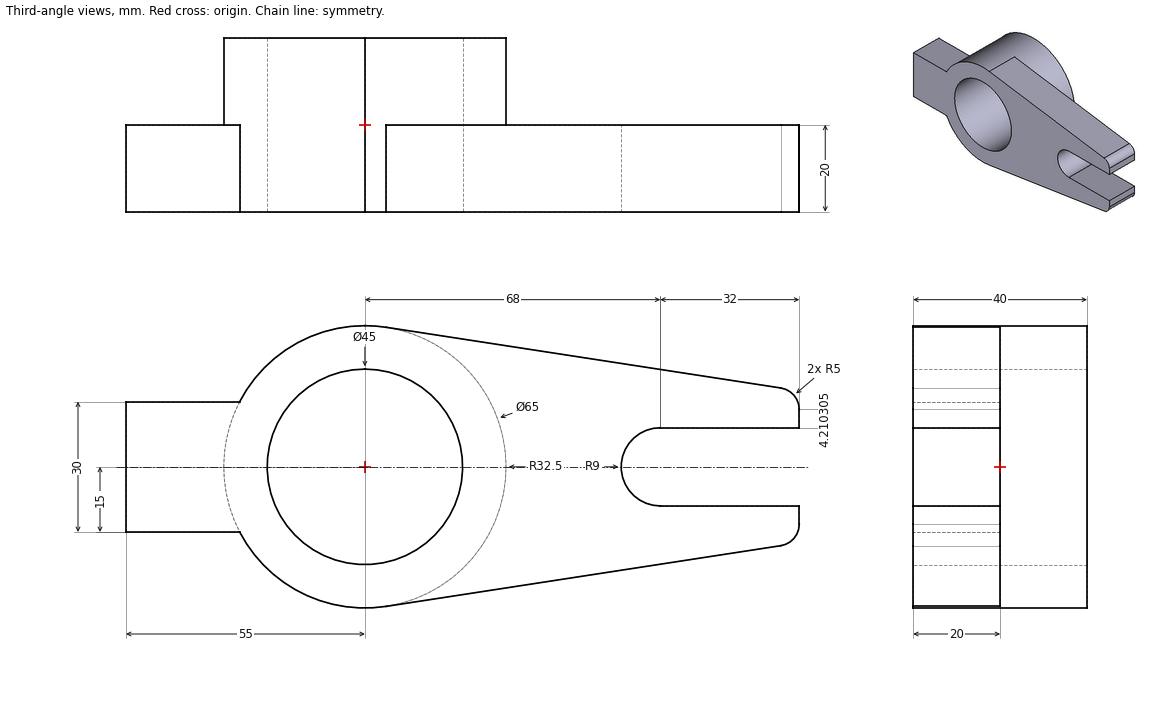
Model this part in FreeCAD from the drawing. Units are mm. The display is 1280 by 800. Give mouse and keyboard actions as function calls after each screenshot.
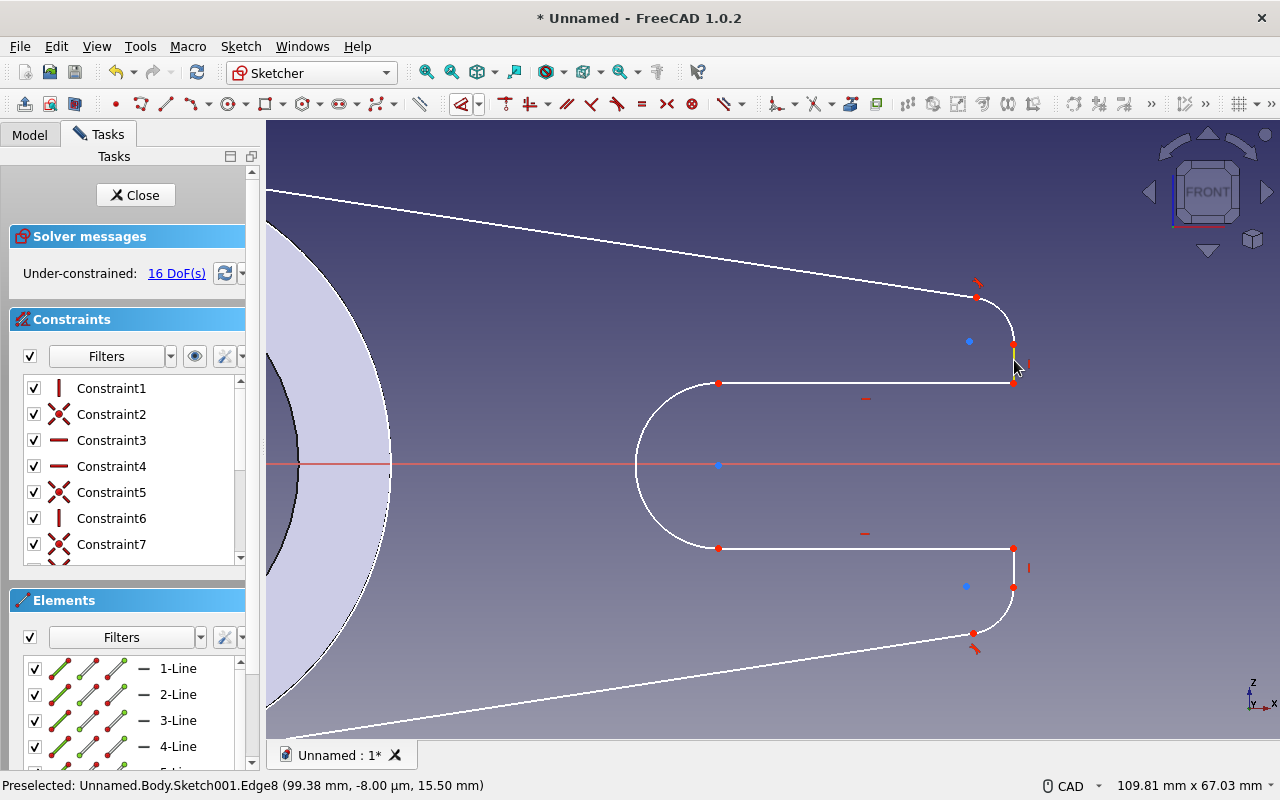
click(1014, 360)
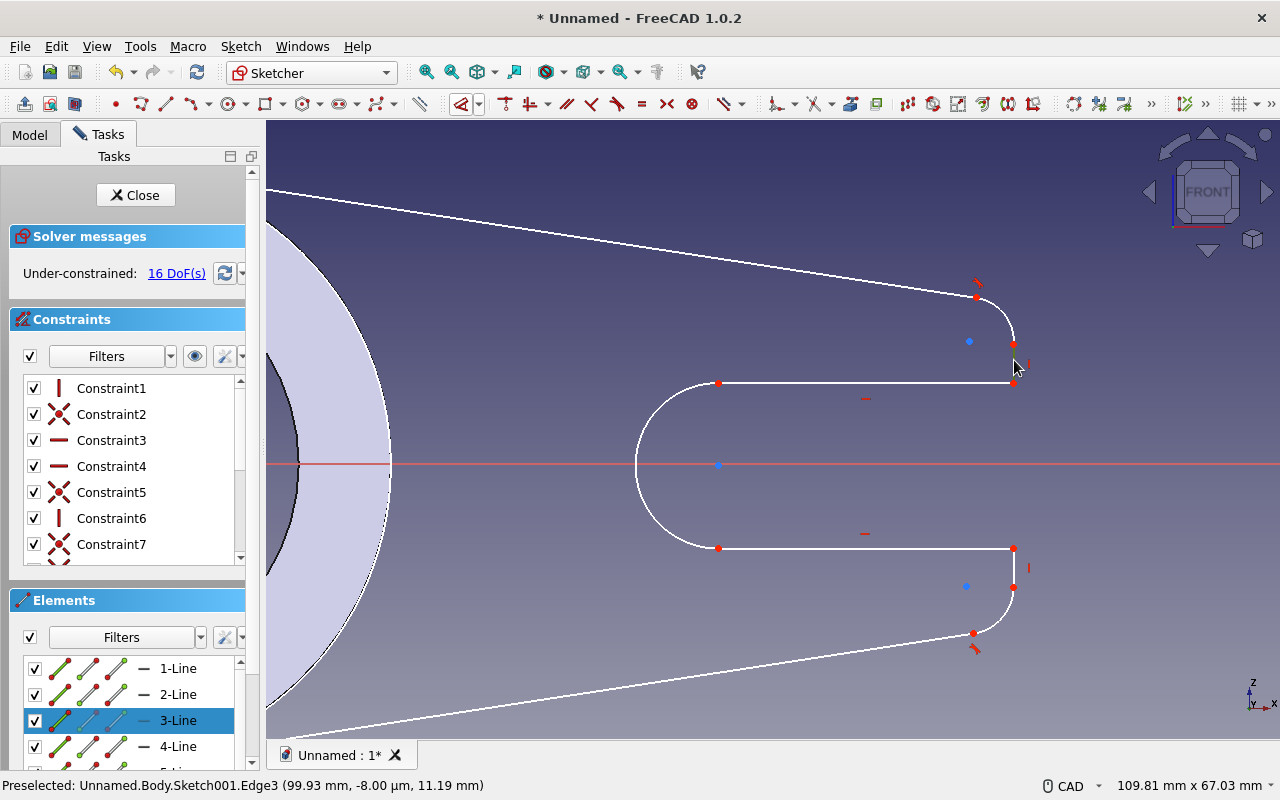
click(1011, 325)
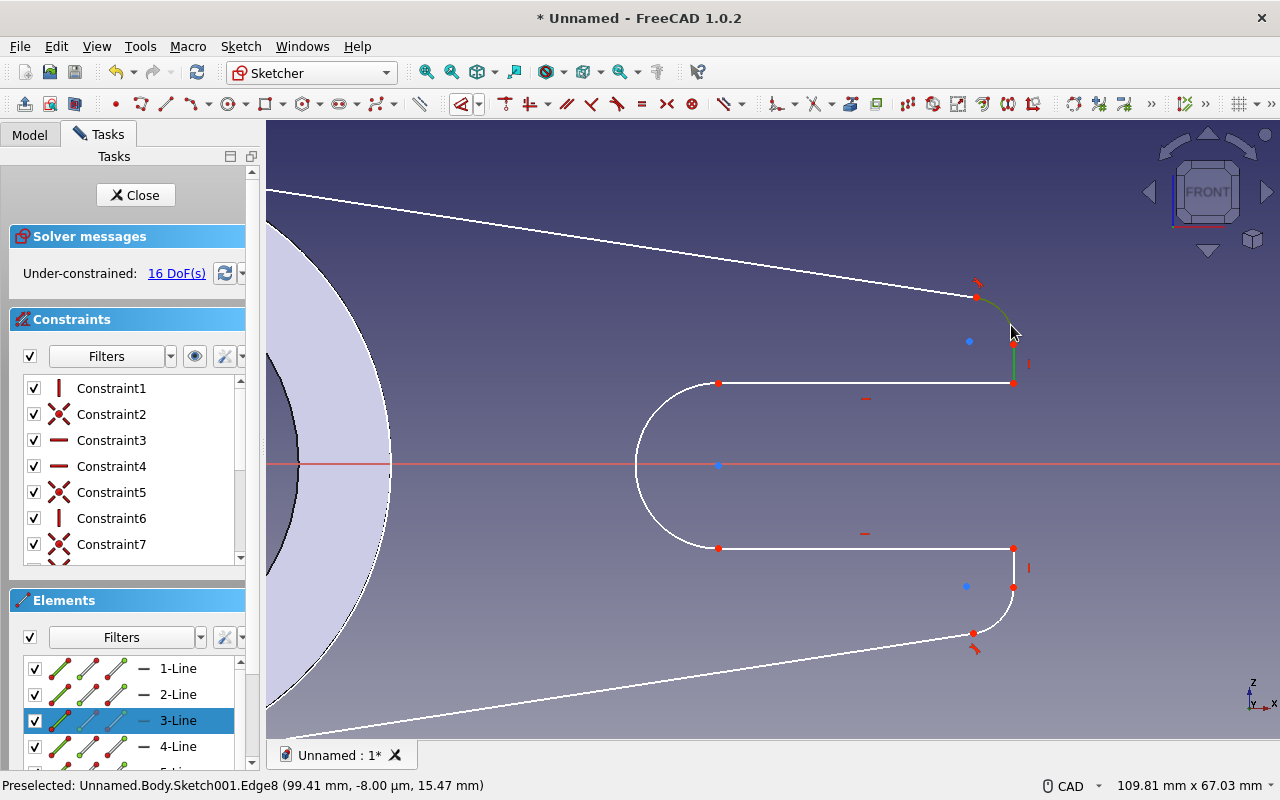
key(t)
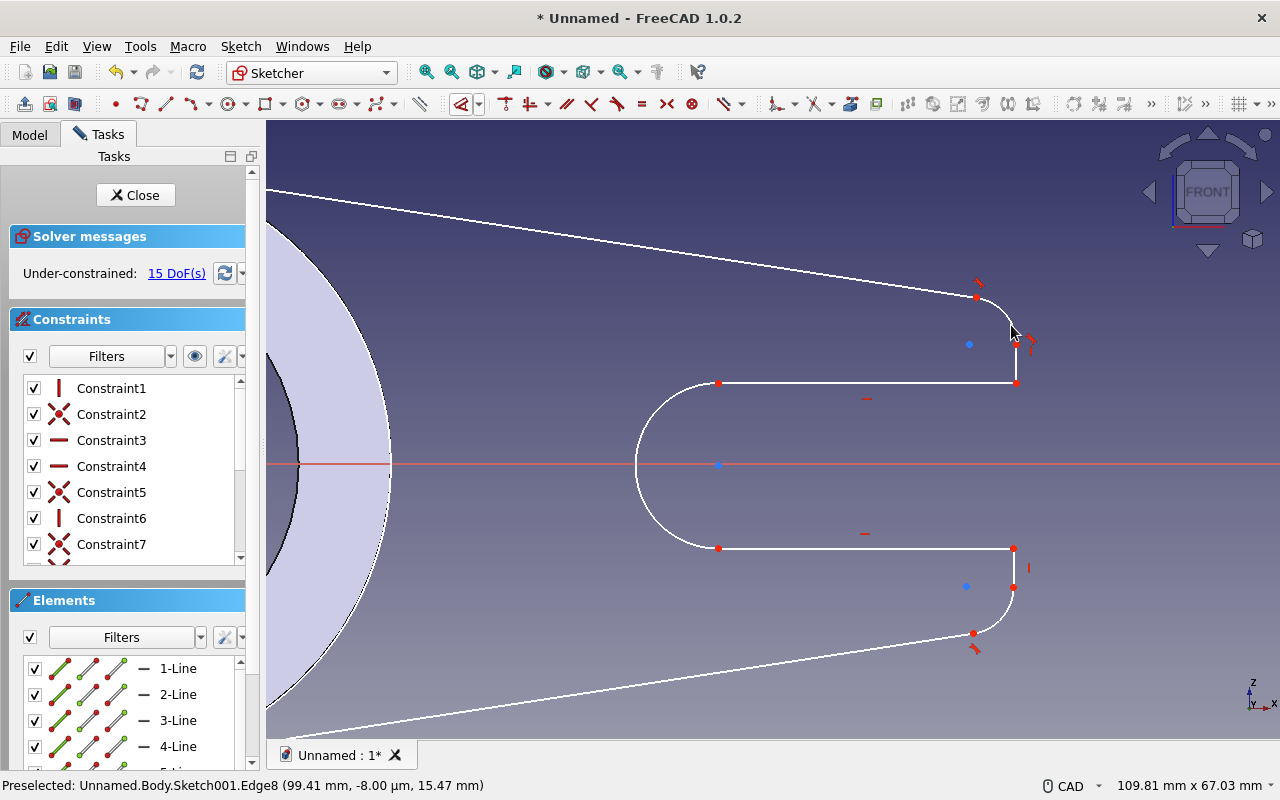
click(927, 383)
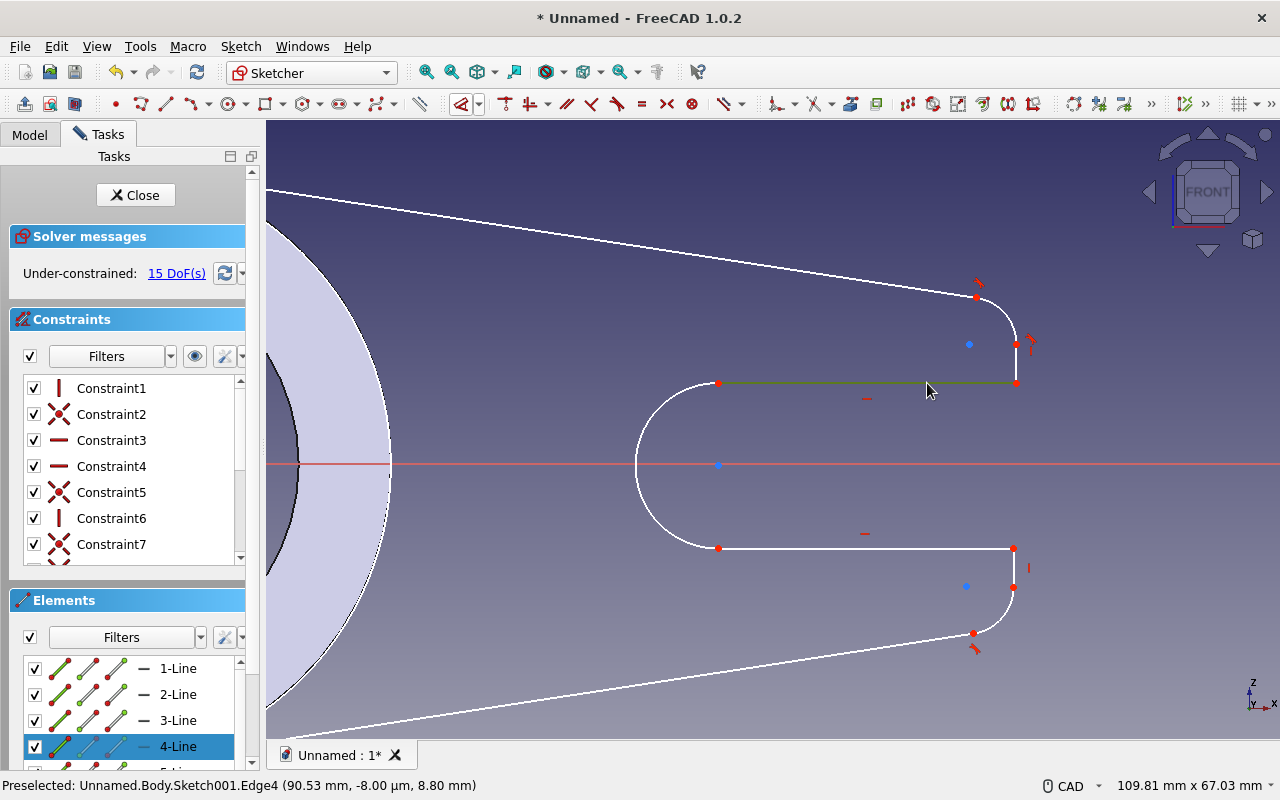
click(651, 417)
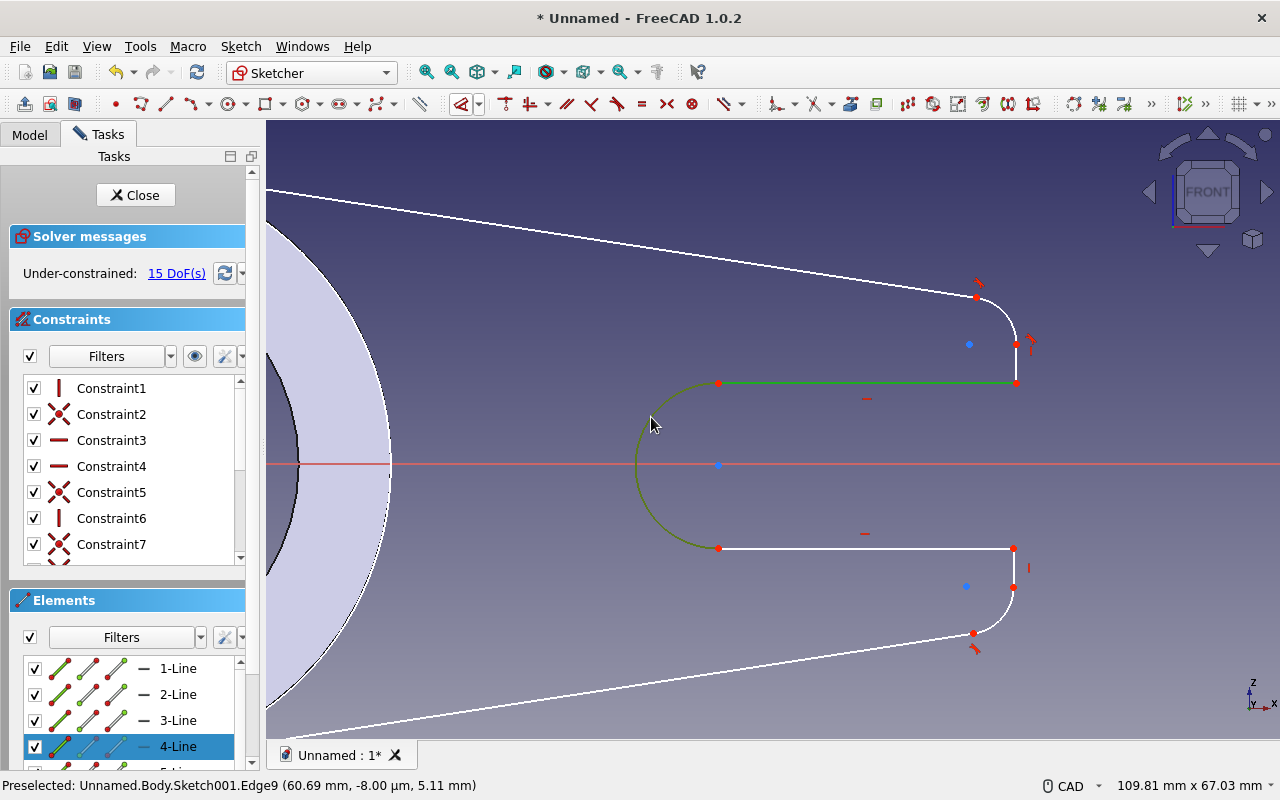
click(617, 104)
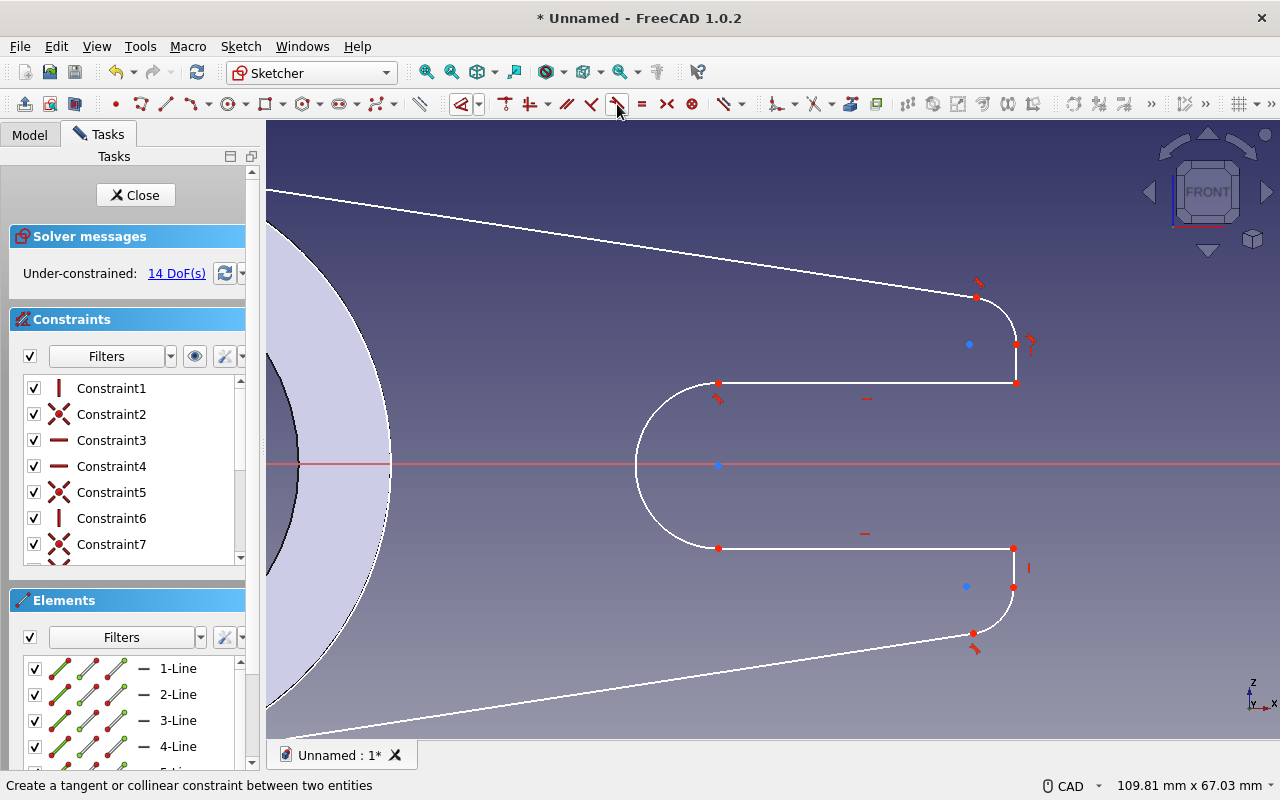
click(807, 549)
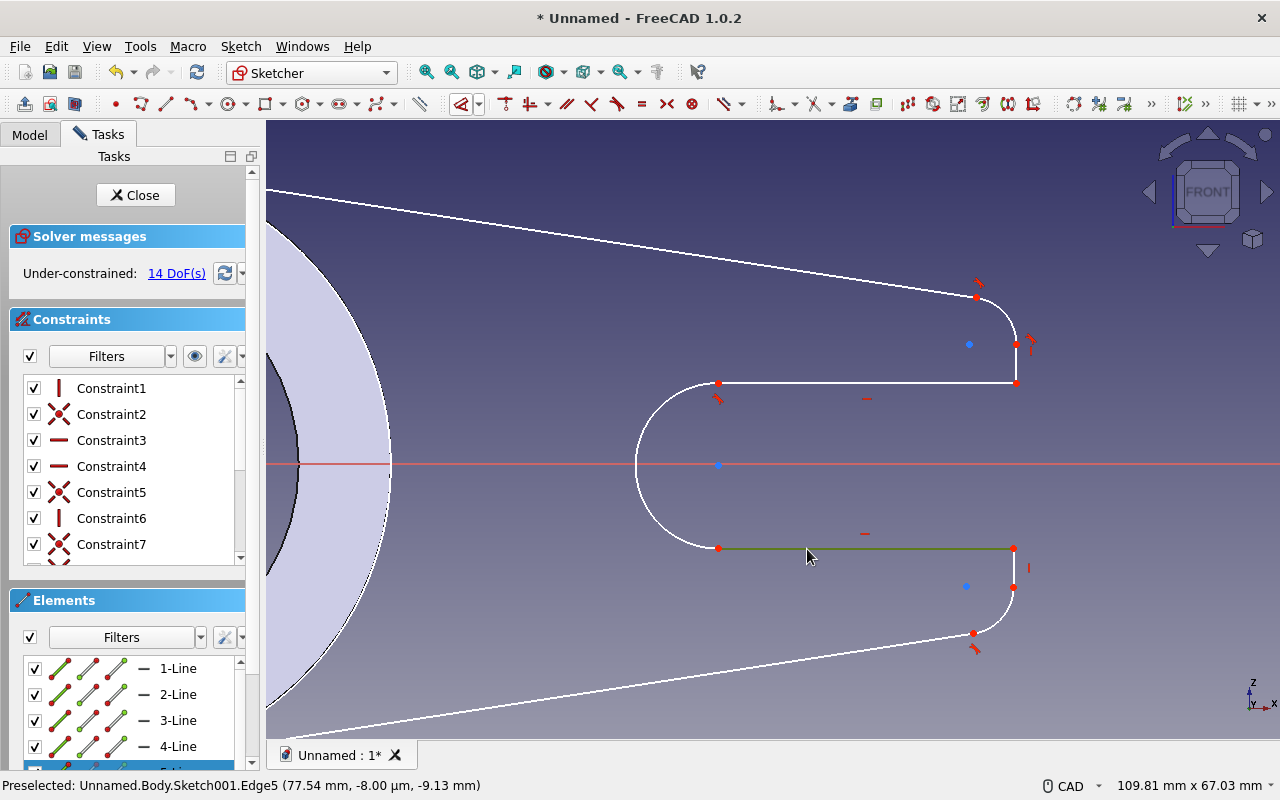
click(651, 417)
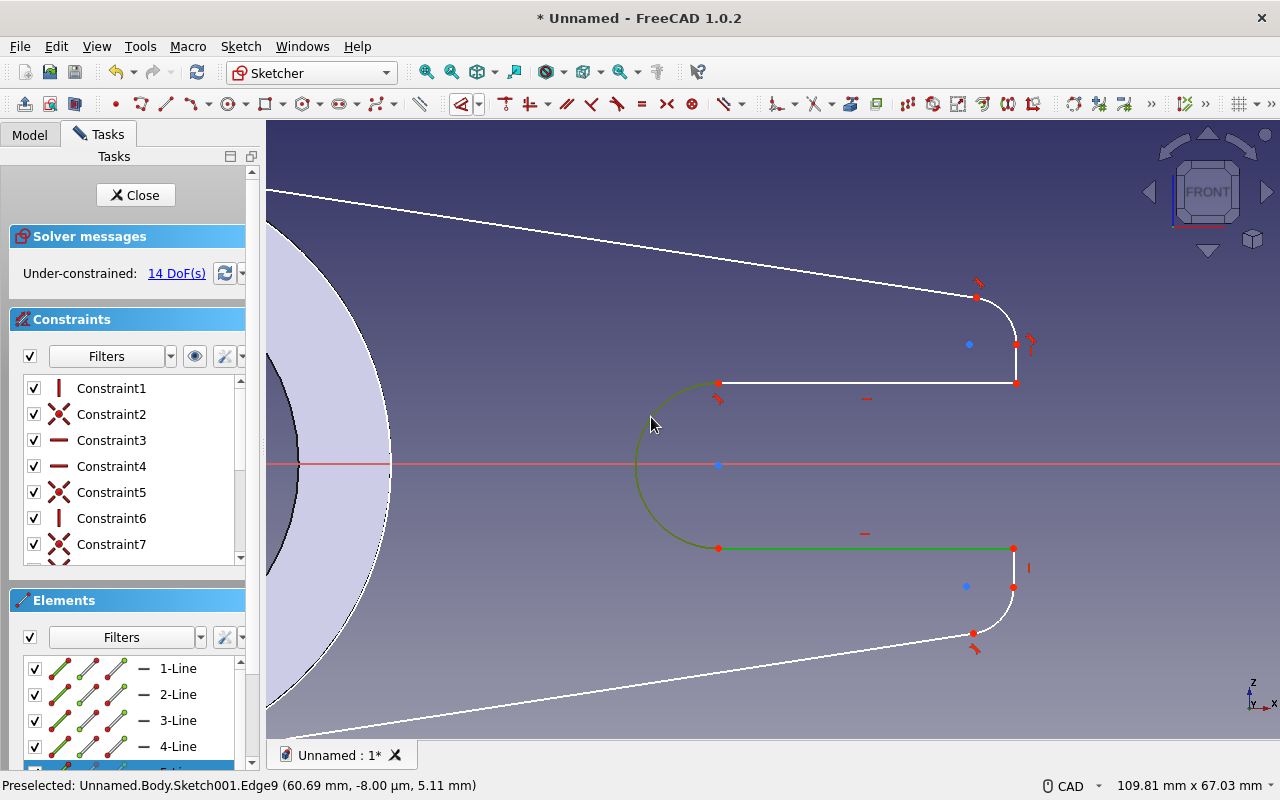
key(t)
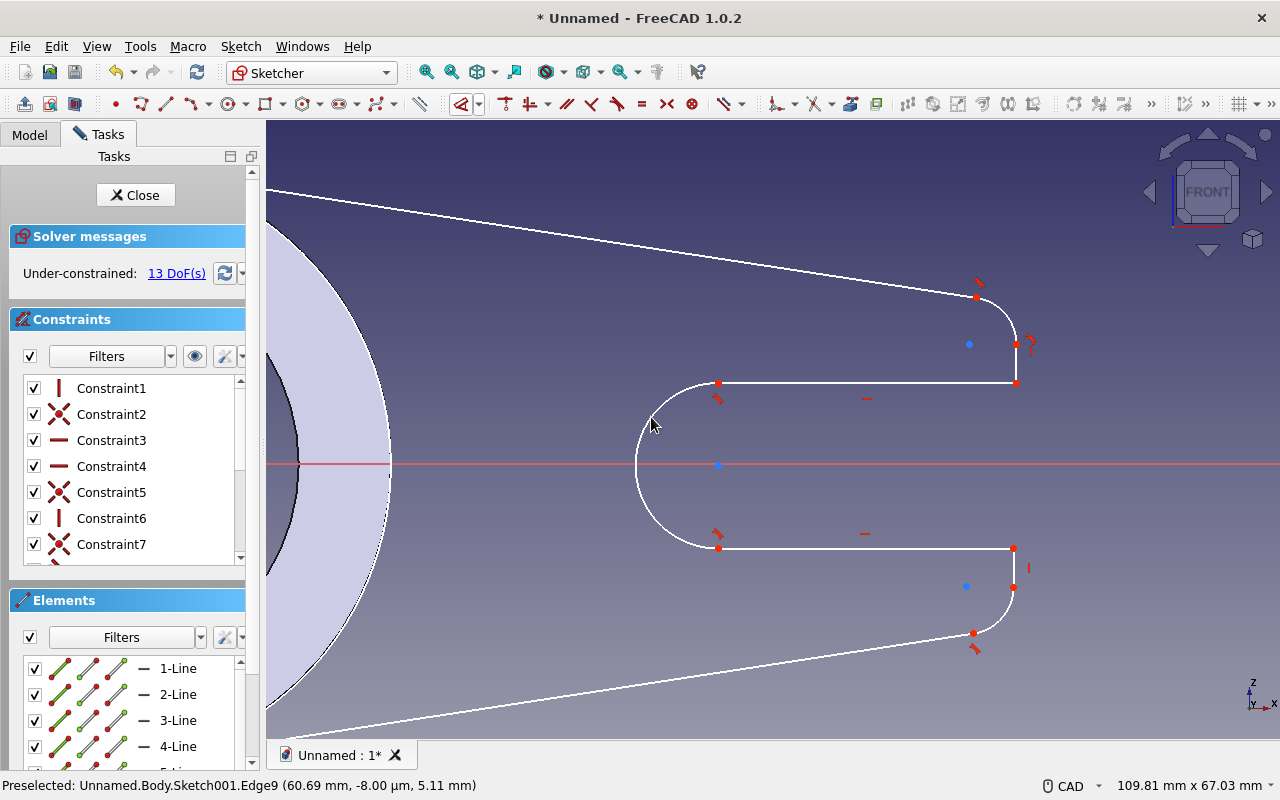
click(1014, 560)